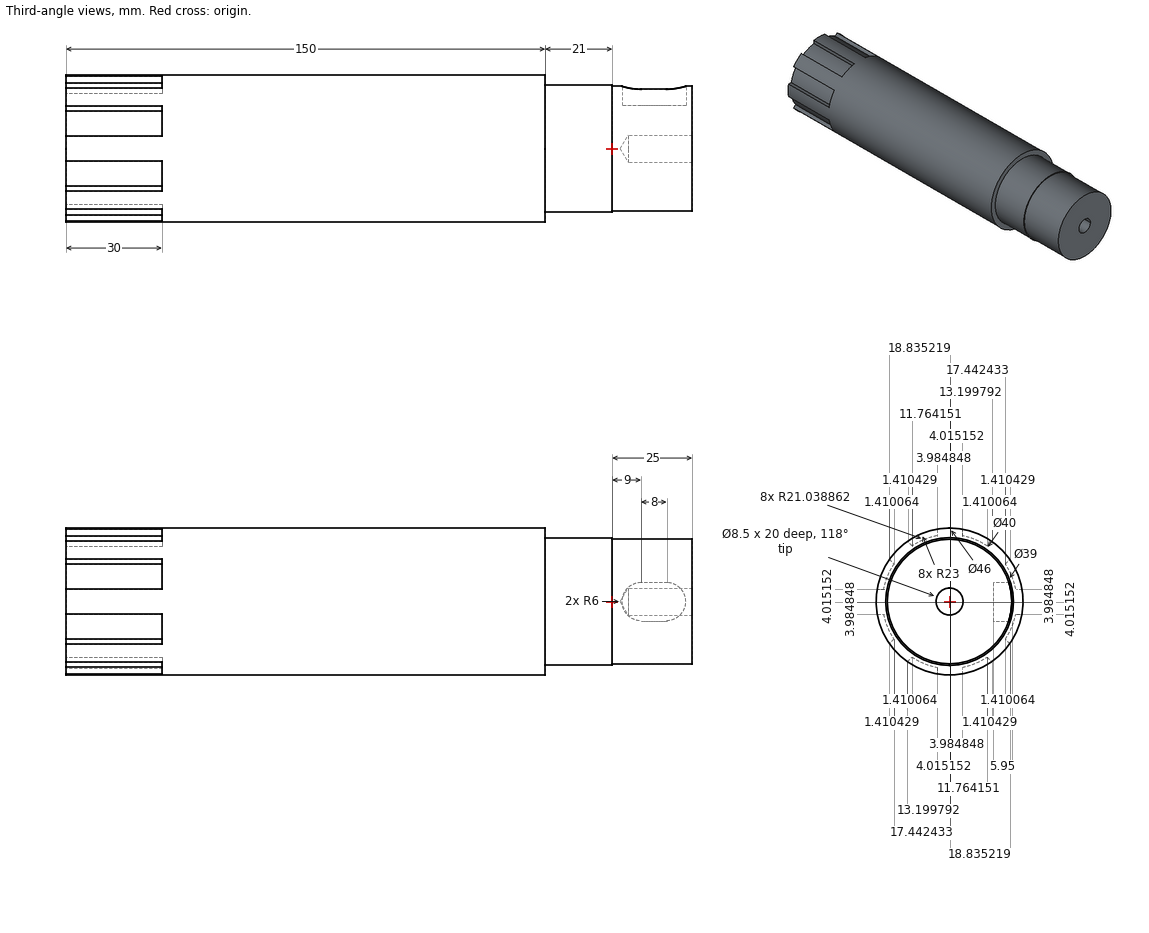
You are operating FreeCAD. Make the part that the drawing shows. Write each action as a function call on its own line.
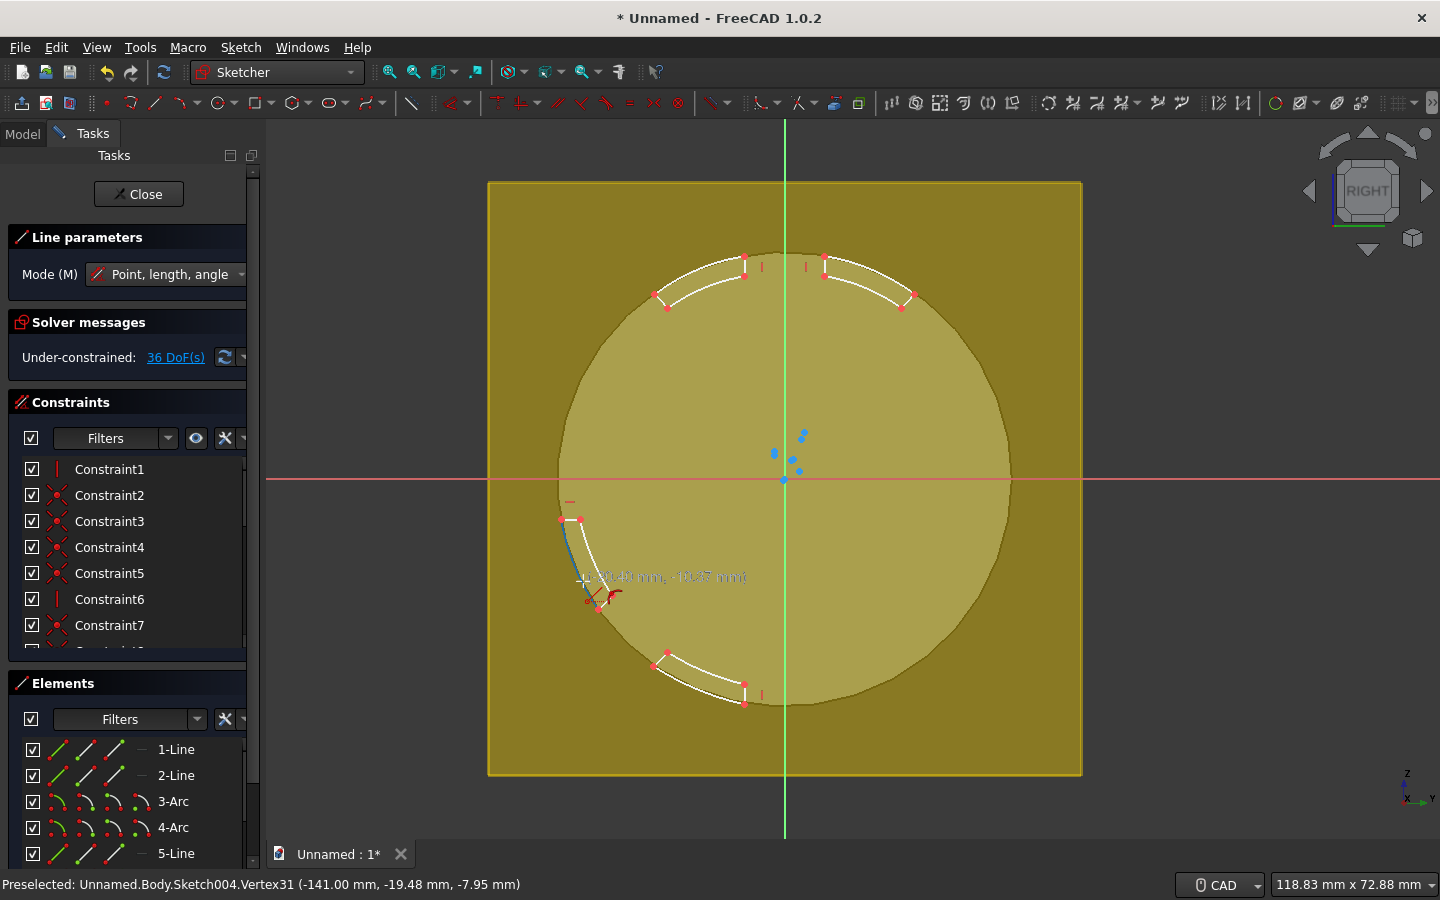
click(599, 349)
click(613, 363)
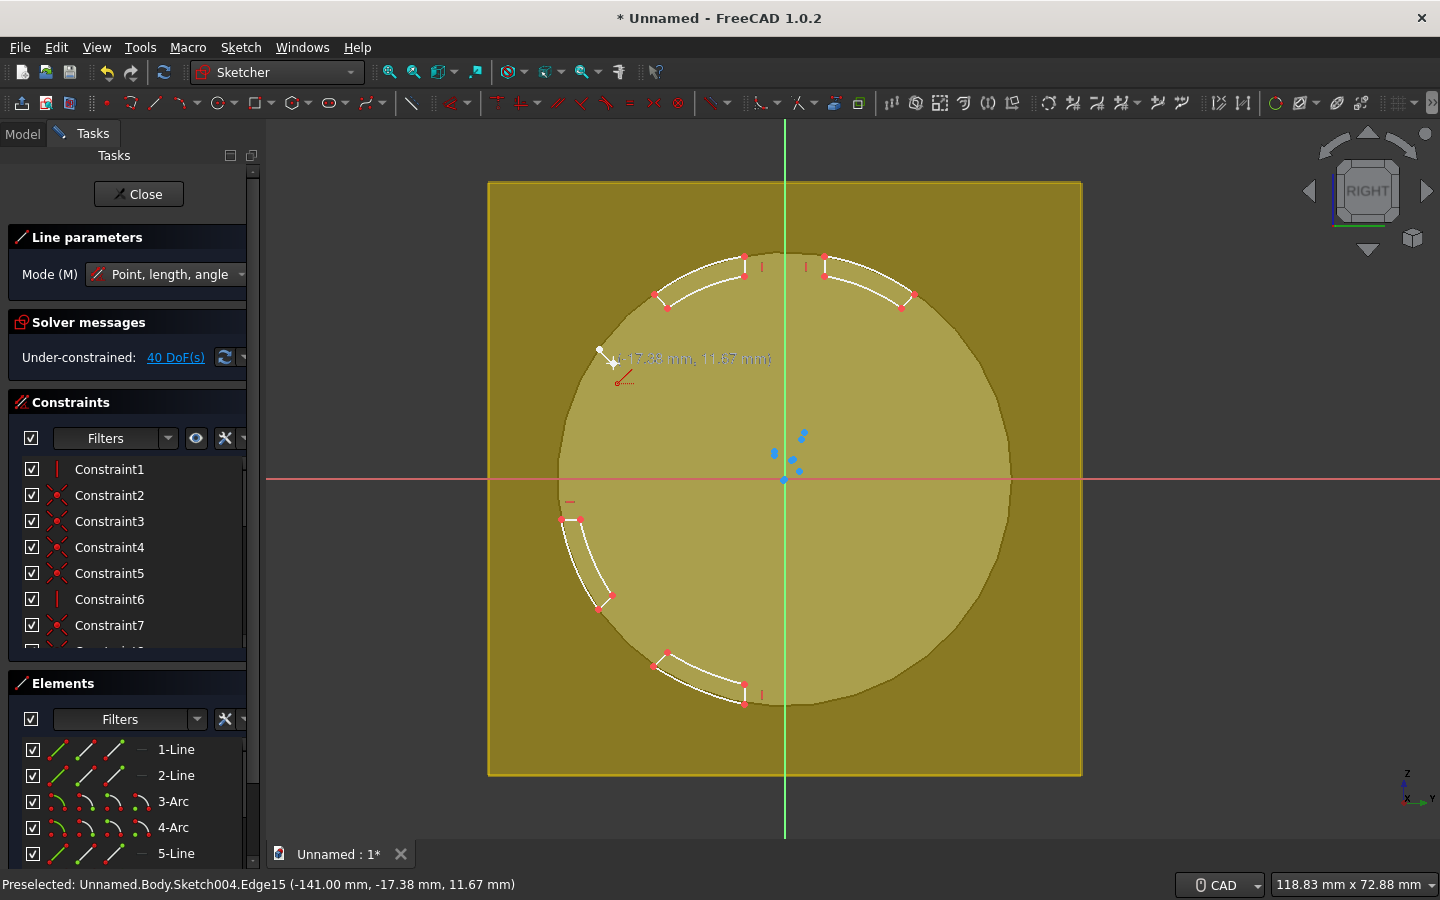
click(581, 440)
click(561, 440)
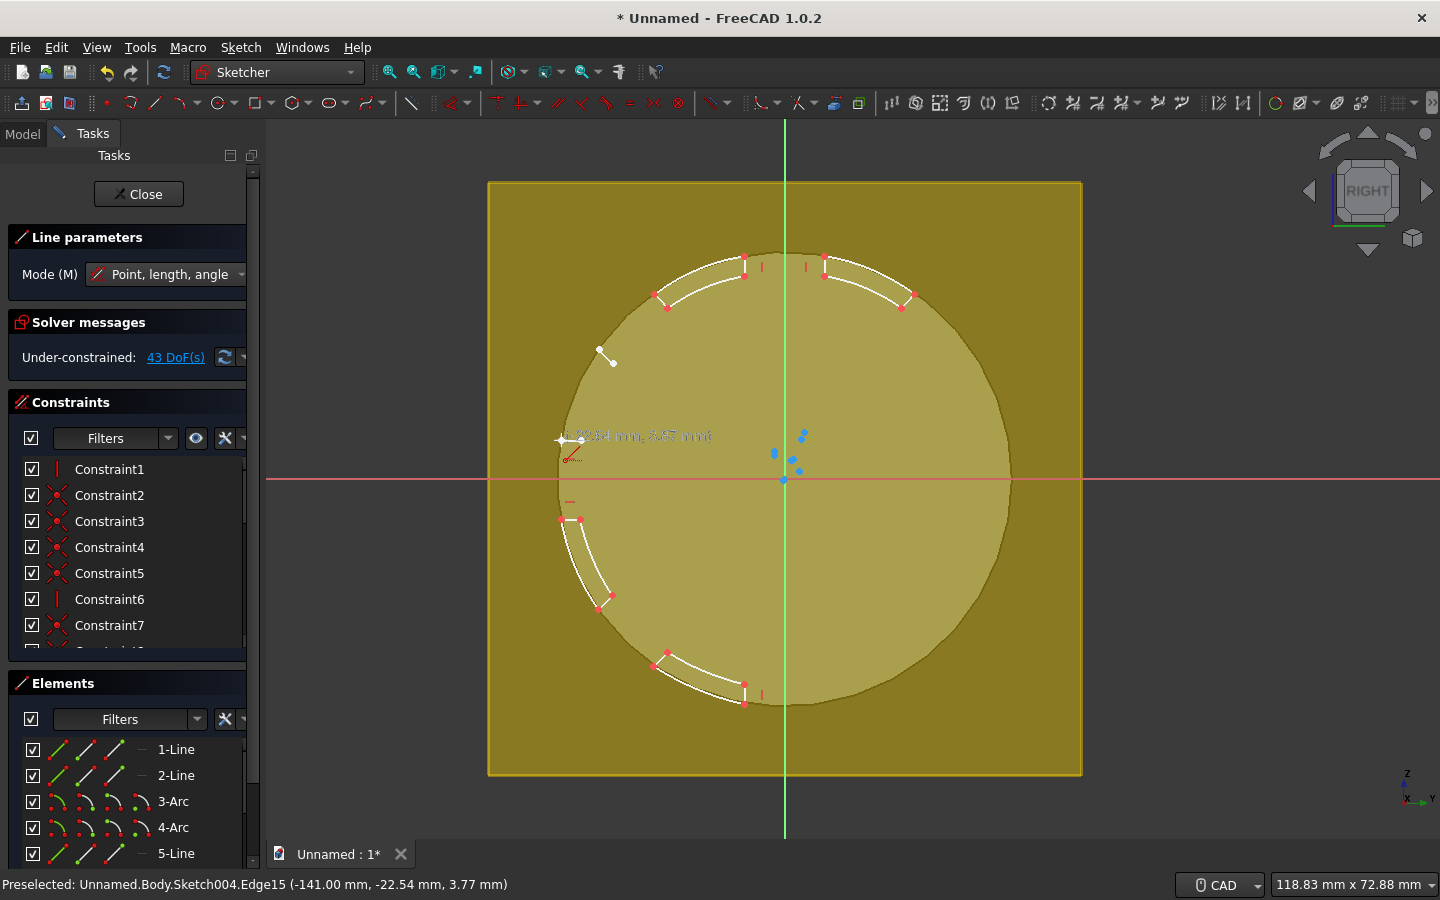
click(180, 104)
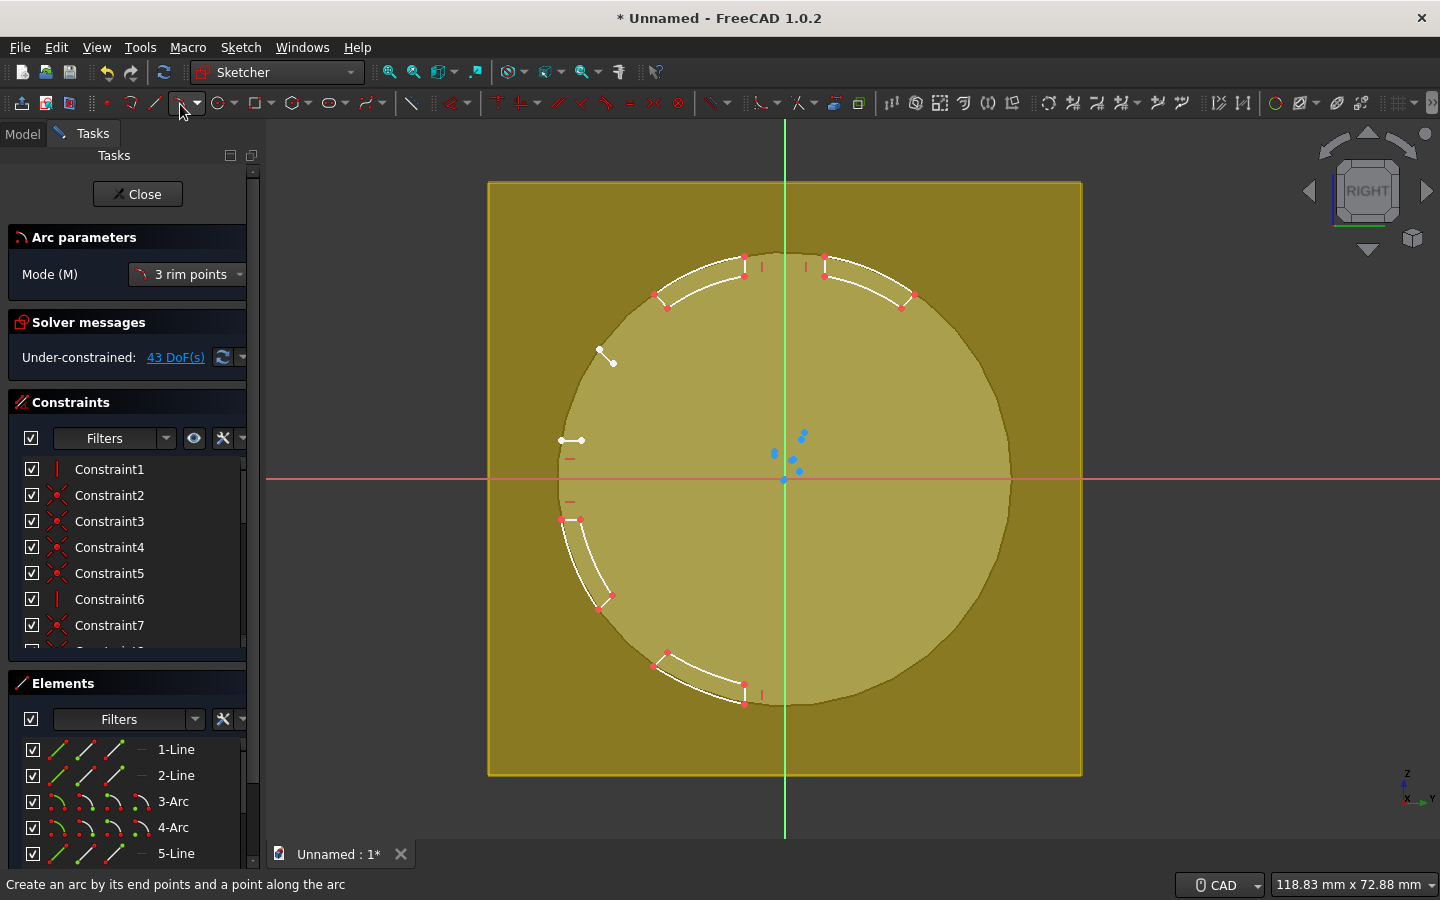
scroll(613, 363, up, 3)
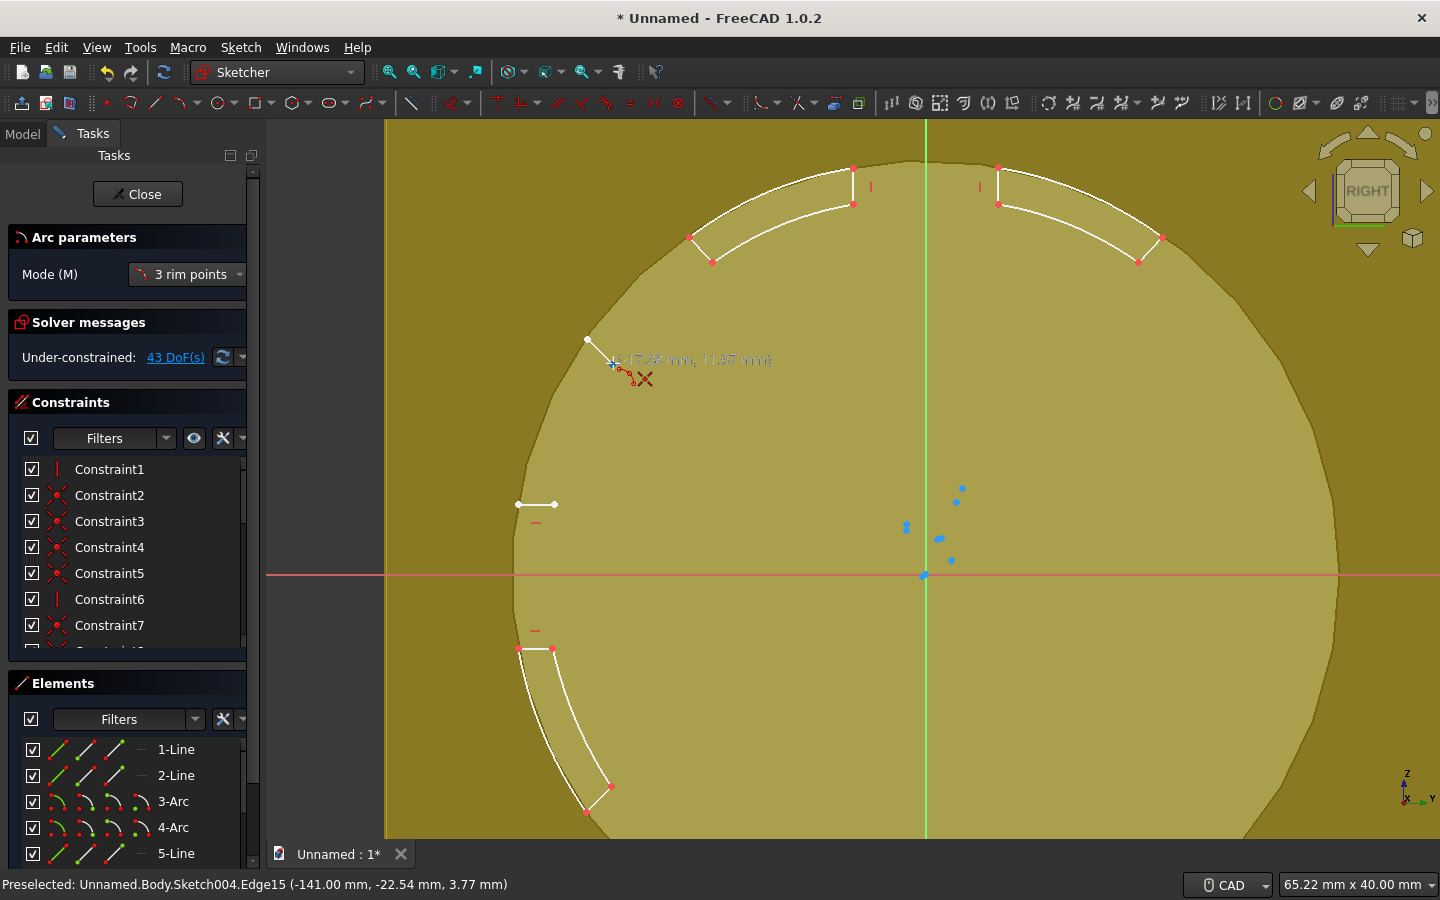
click(613, 365)
click(554, 505)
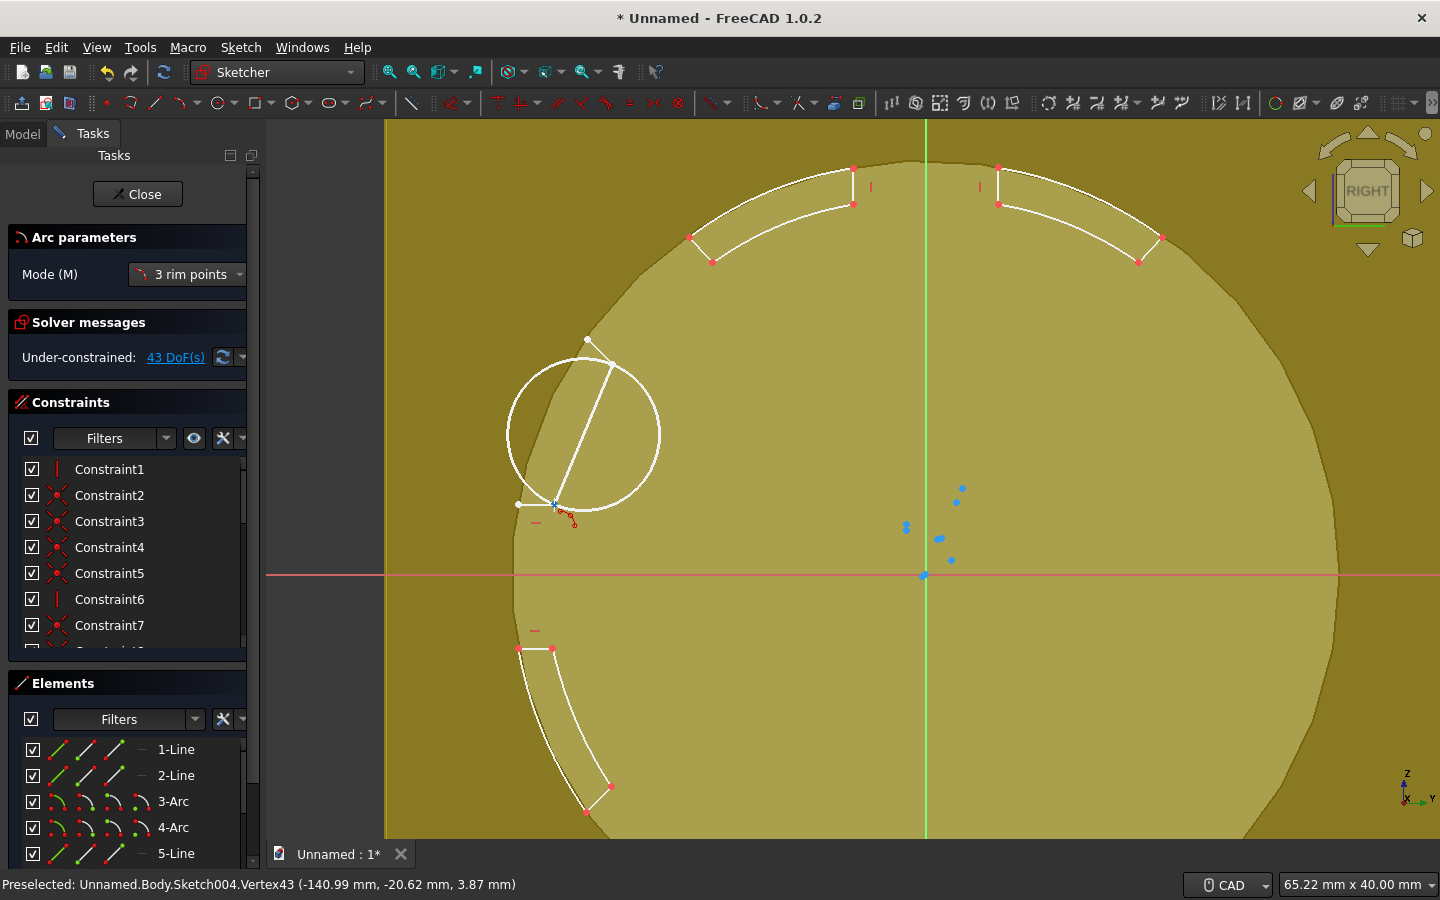
scroll(576, 429, up, 4)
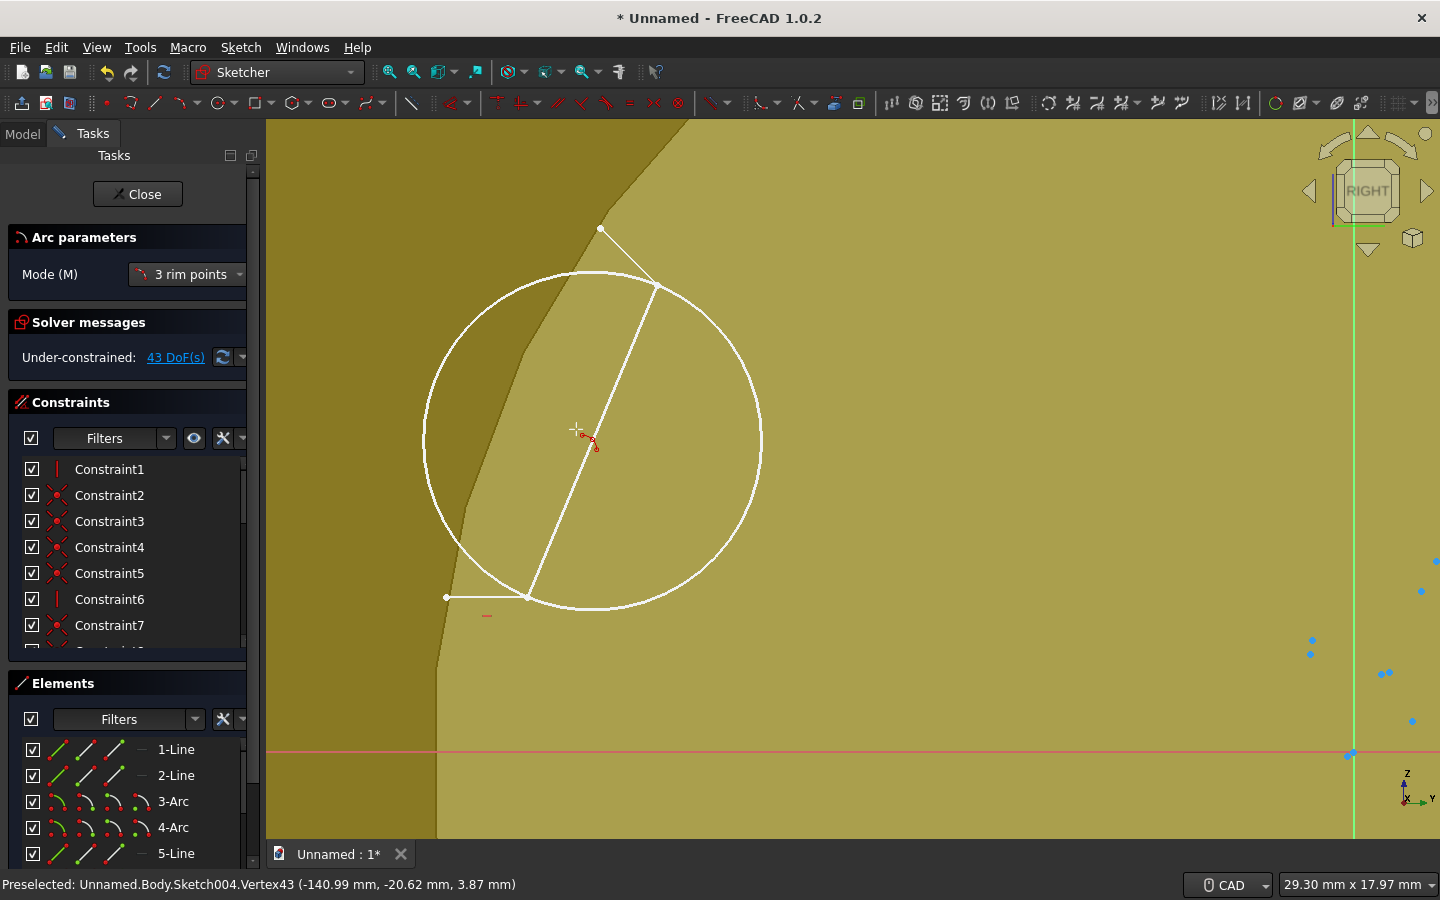
click(575, 429)